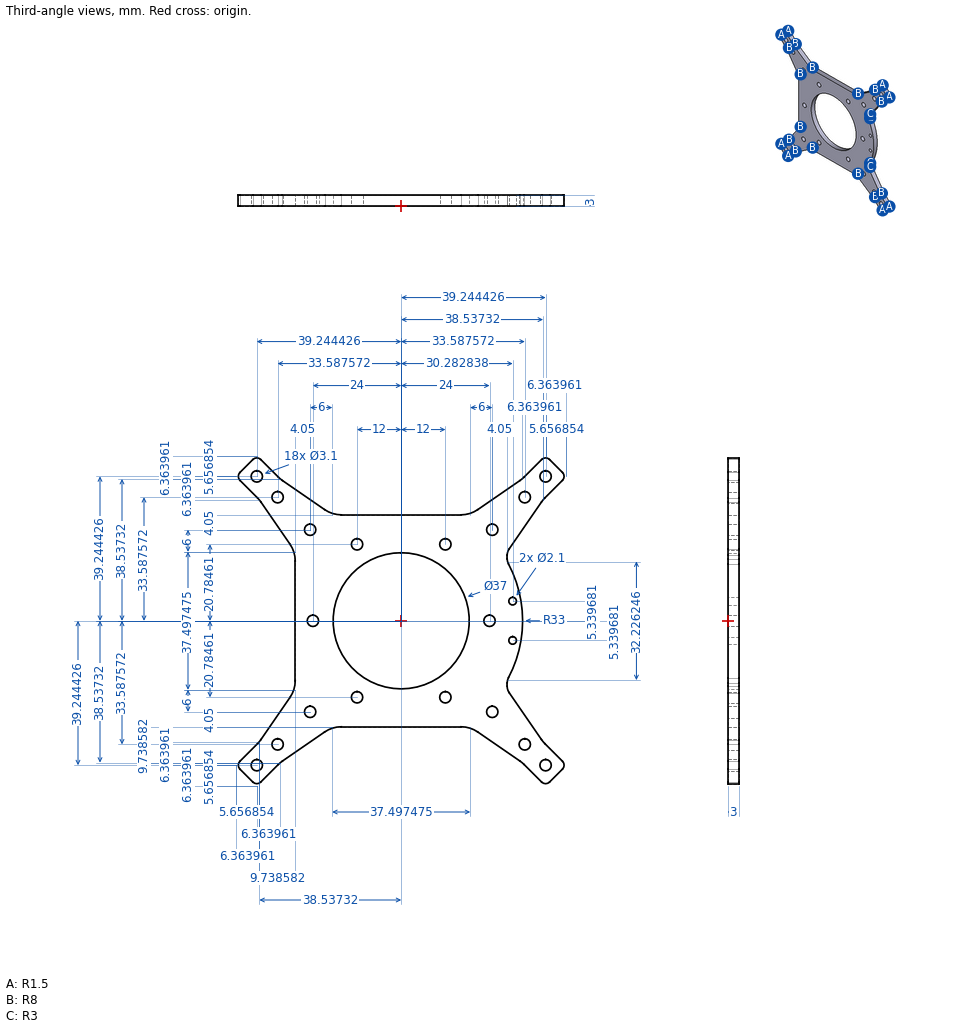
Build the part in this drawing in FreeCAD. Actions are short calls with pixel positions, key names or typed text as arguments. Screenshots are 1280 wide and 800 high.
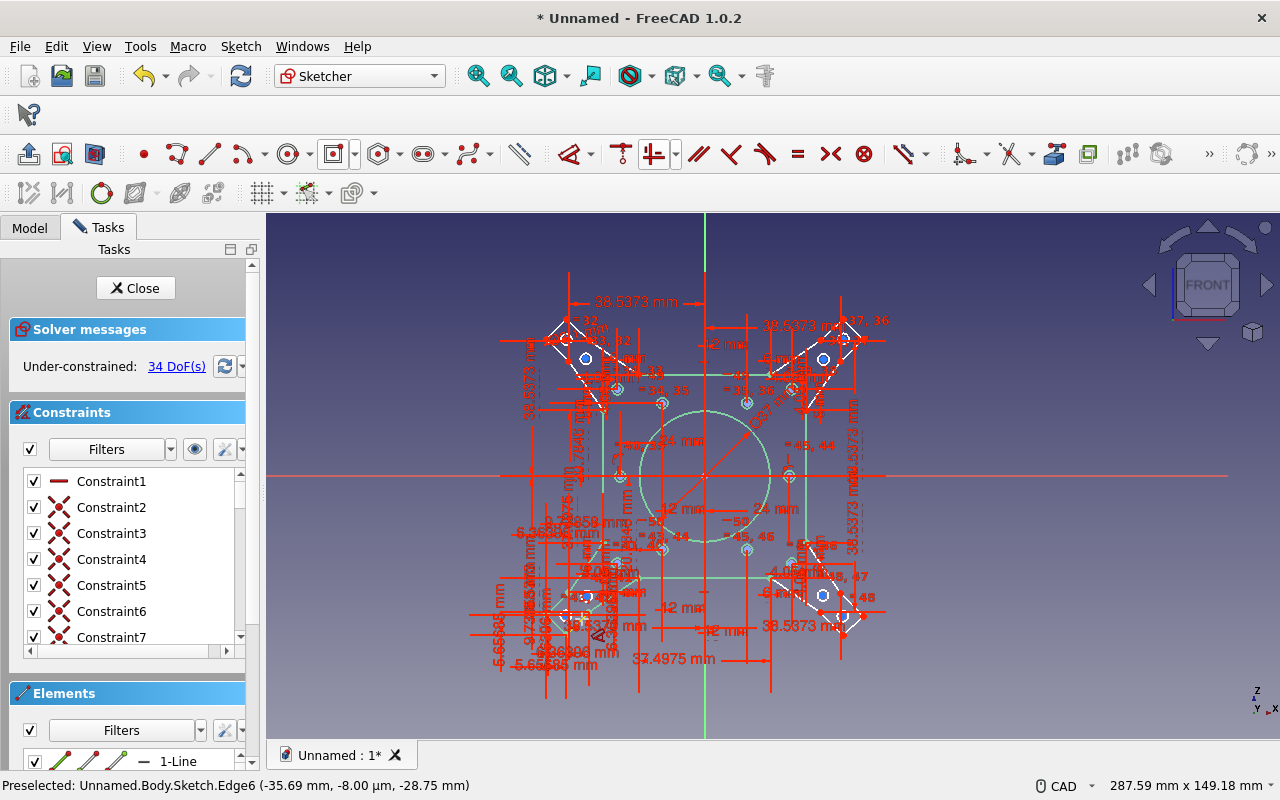
scroll(562, 355, up, 3)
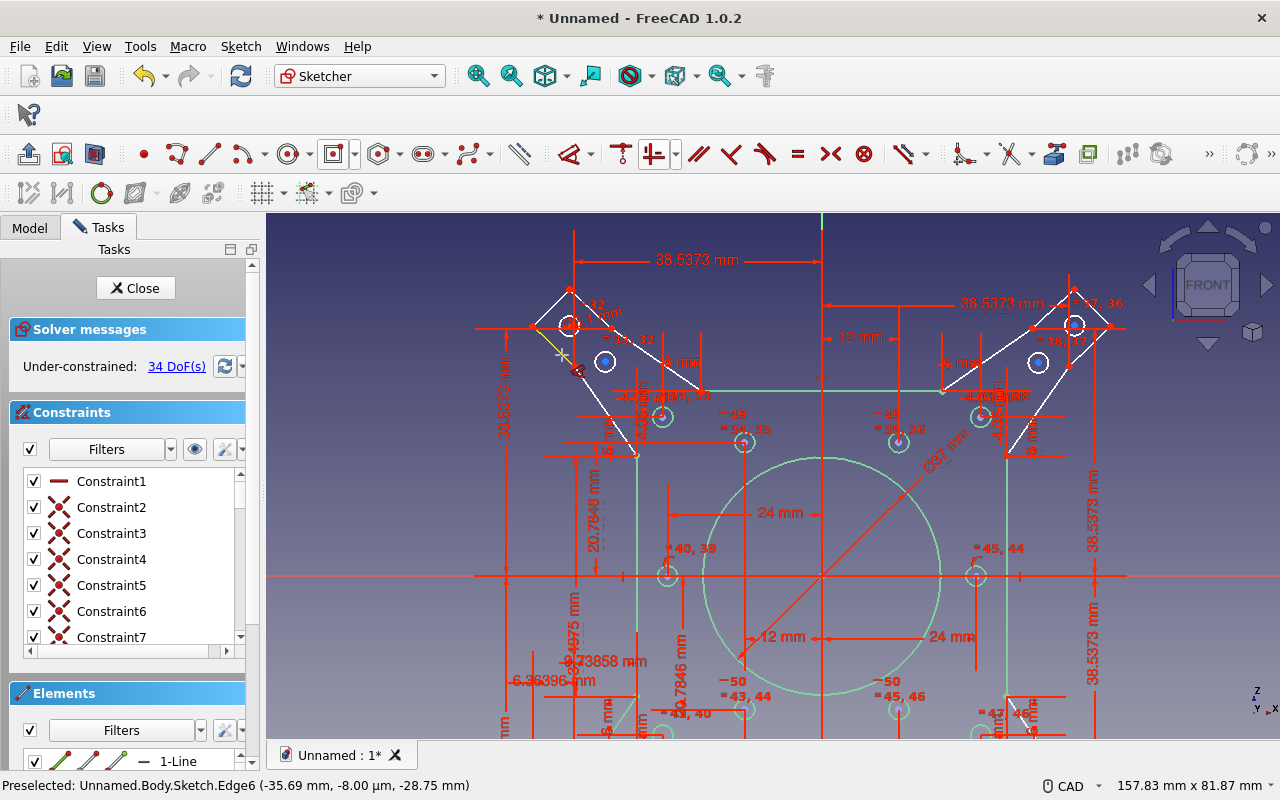
click(562, 354)
click(544, 292)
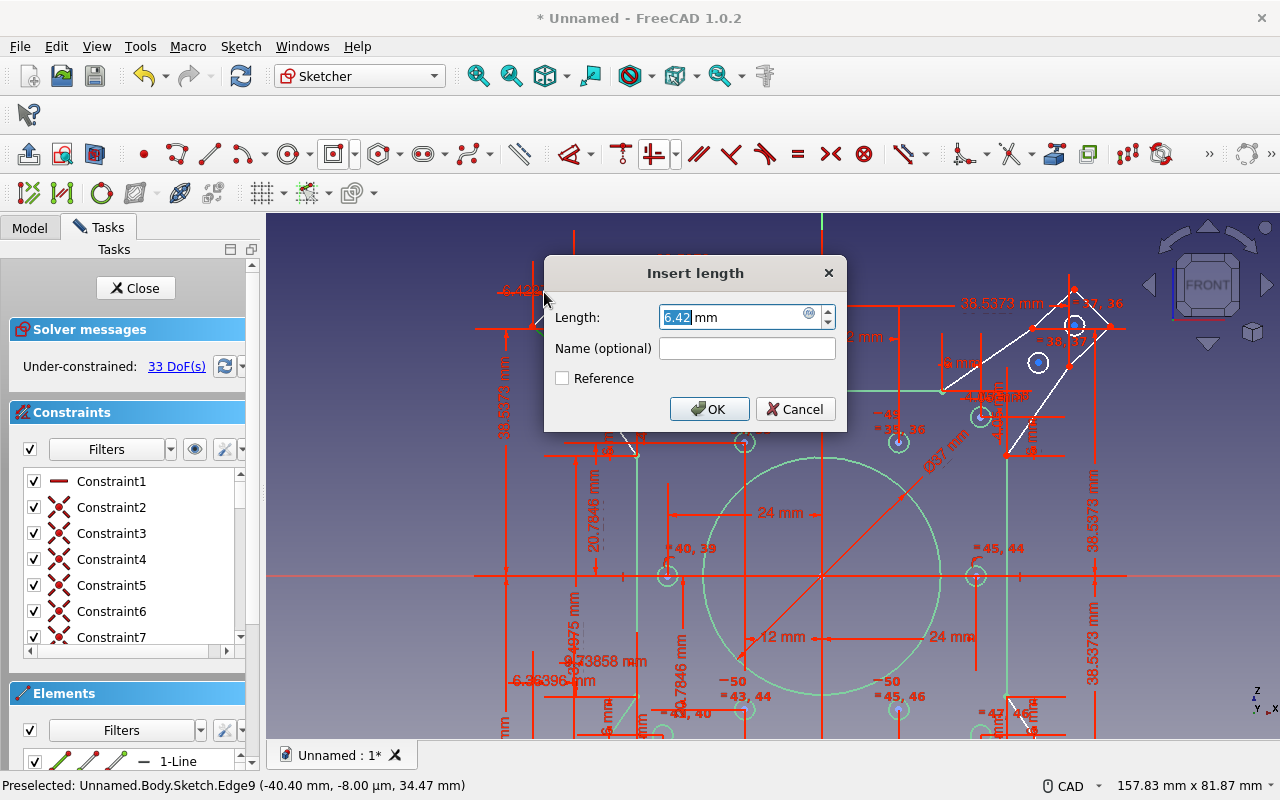
text(6.363961)
key(Return)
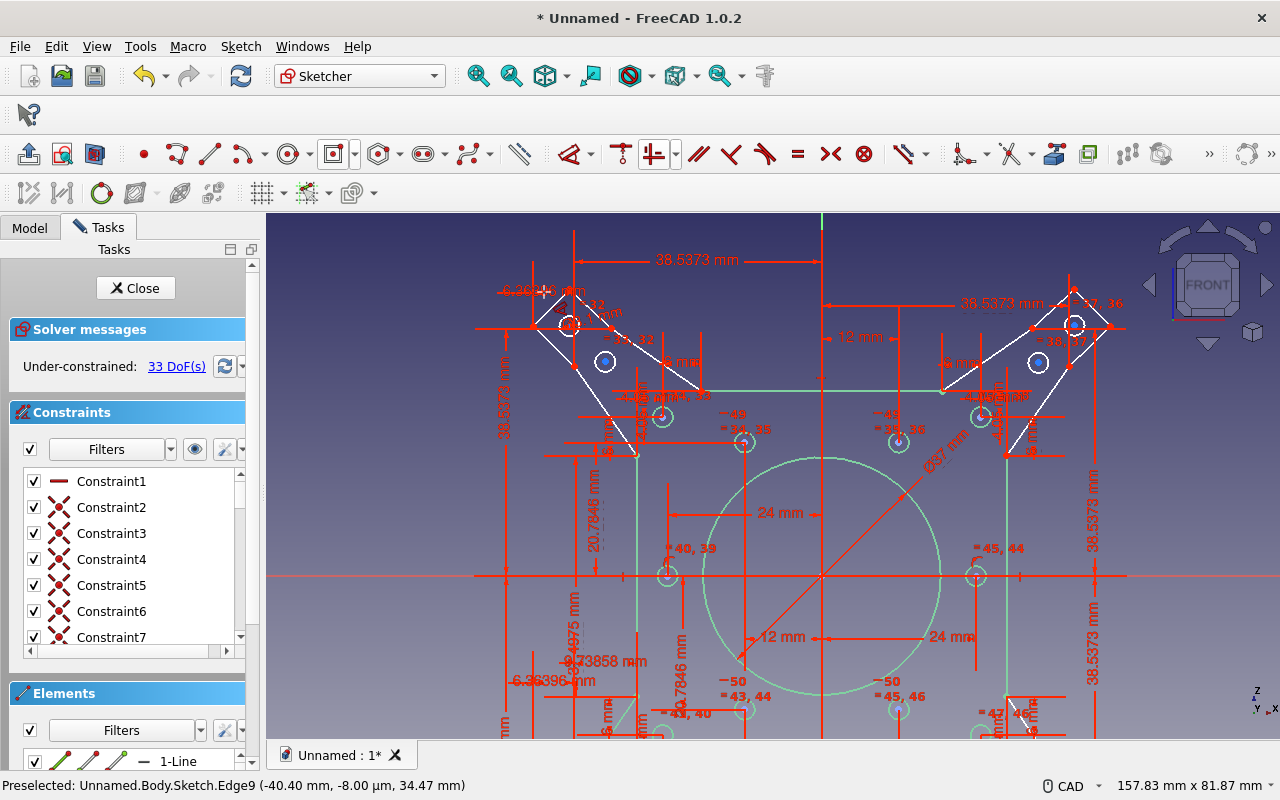
click(562, 354)
click(499, 346)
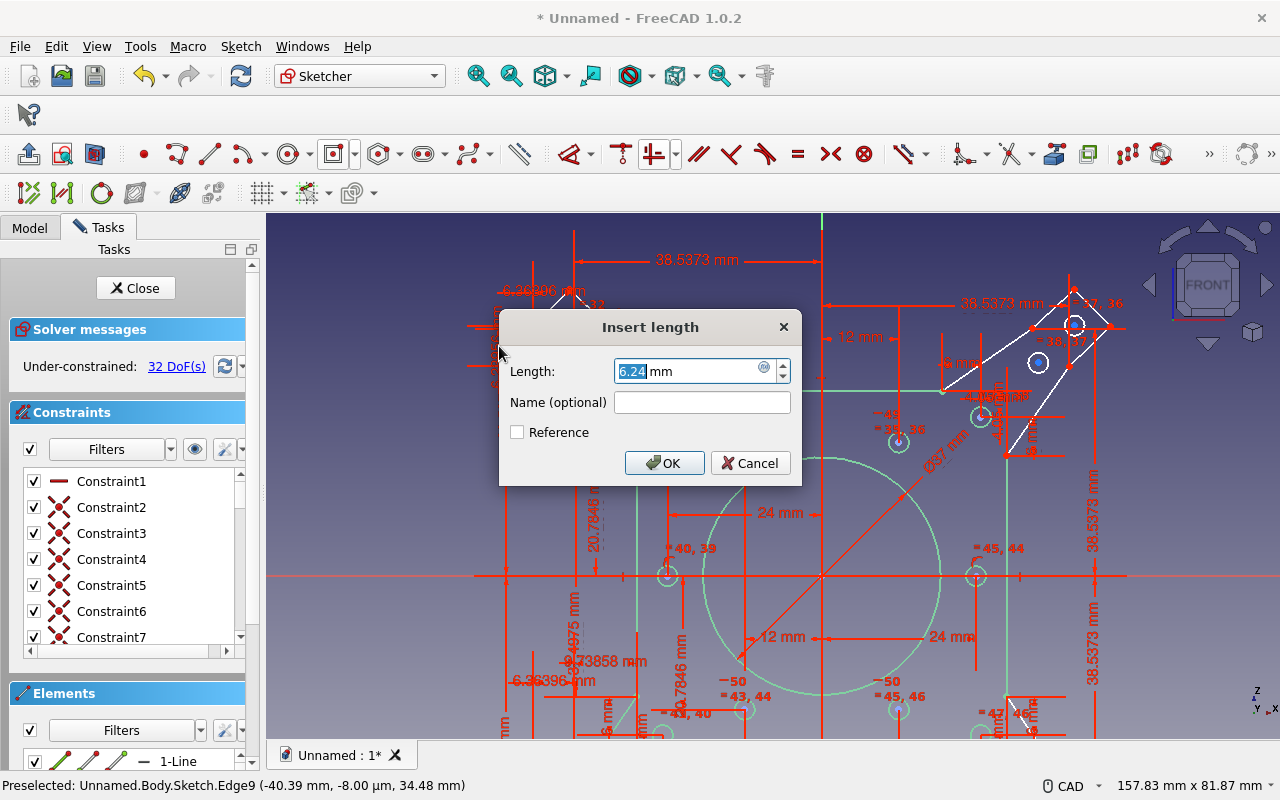
text(6.363961)
key(Return)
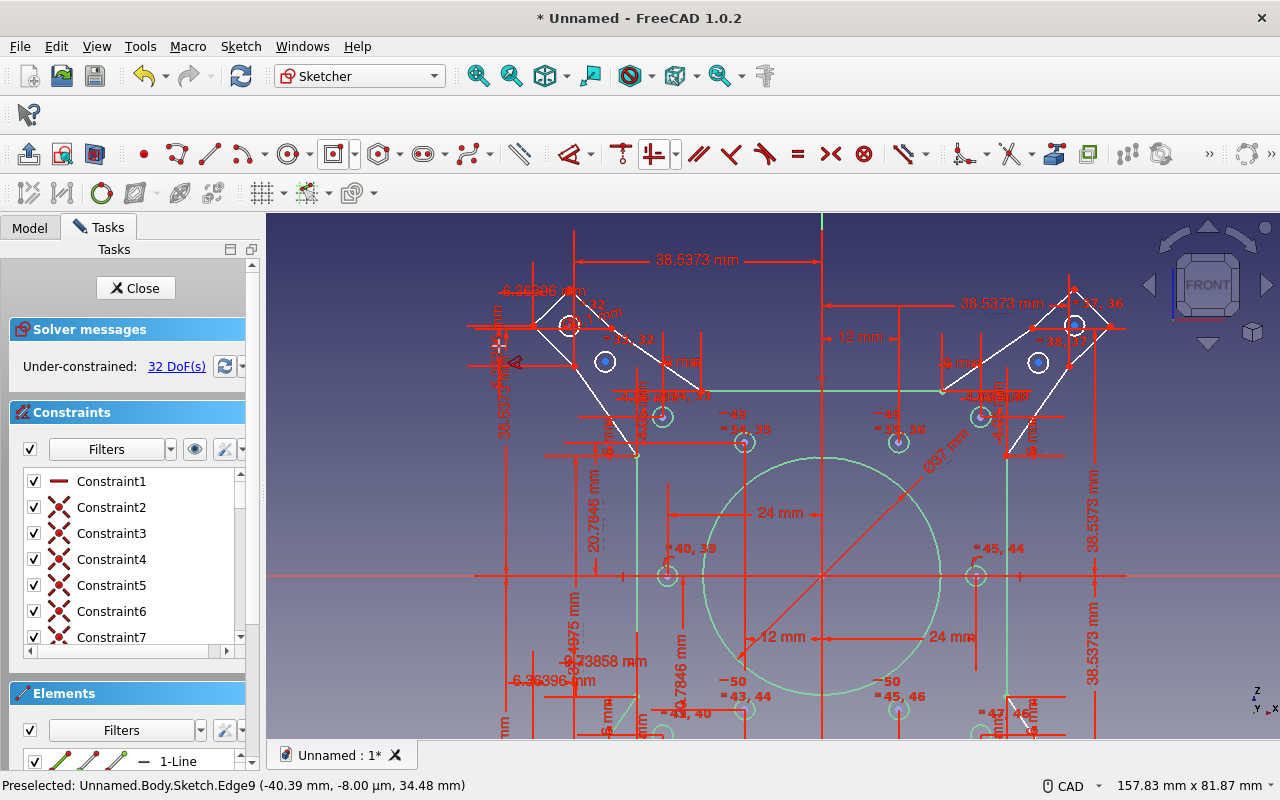
click(544, 315)
click(551, 256)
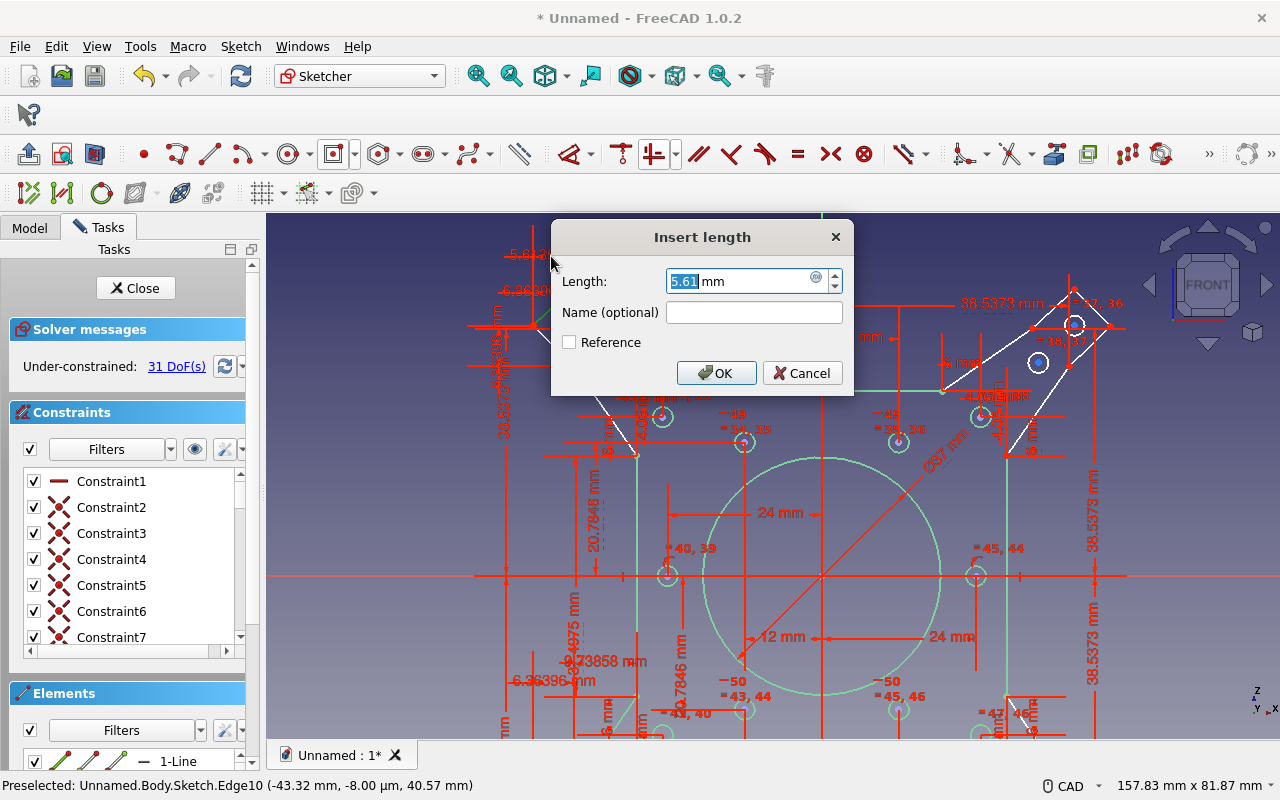
text(5.656854)
key(Return)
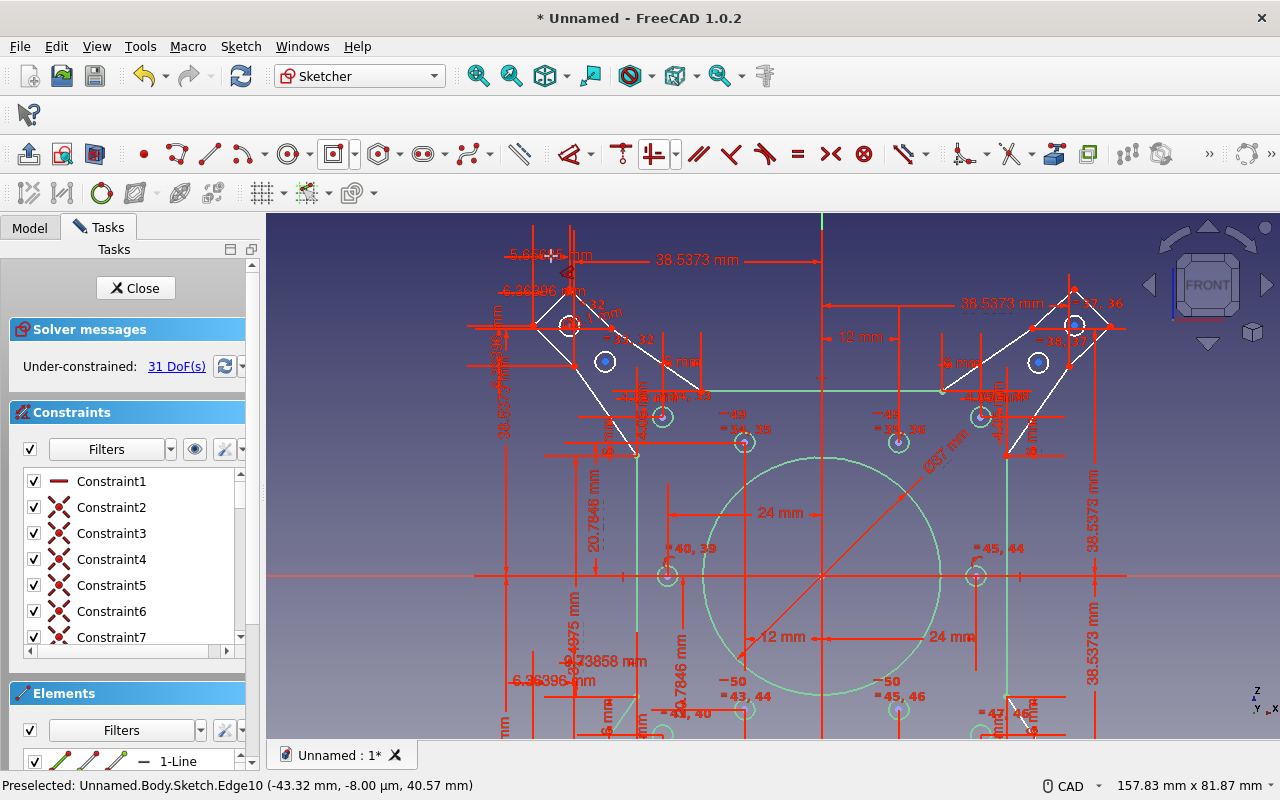
click(544, 315)
click(499, 316)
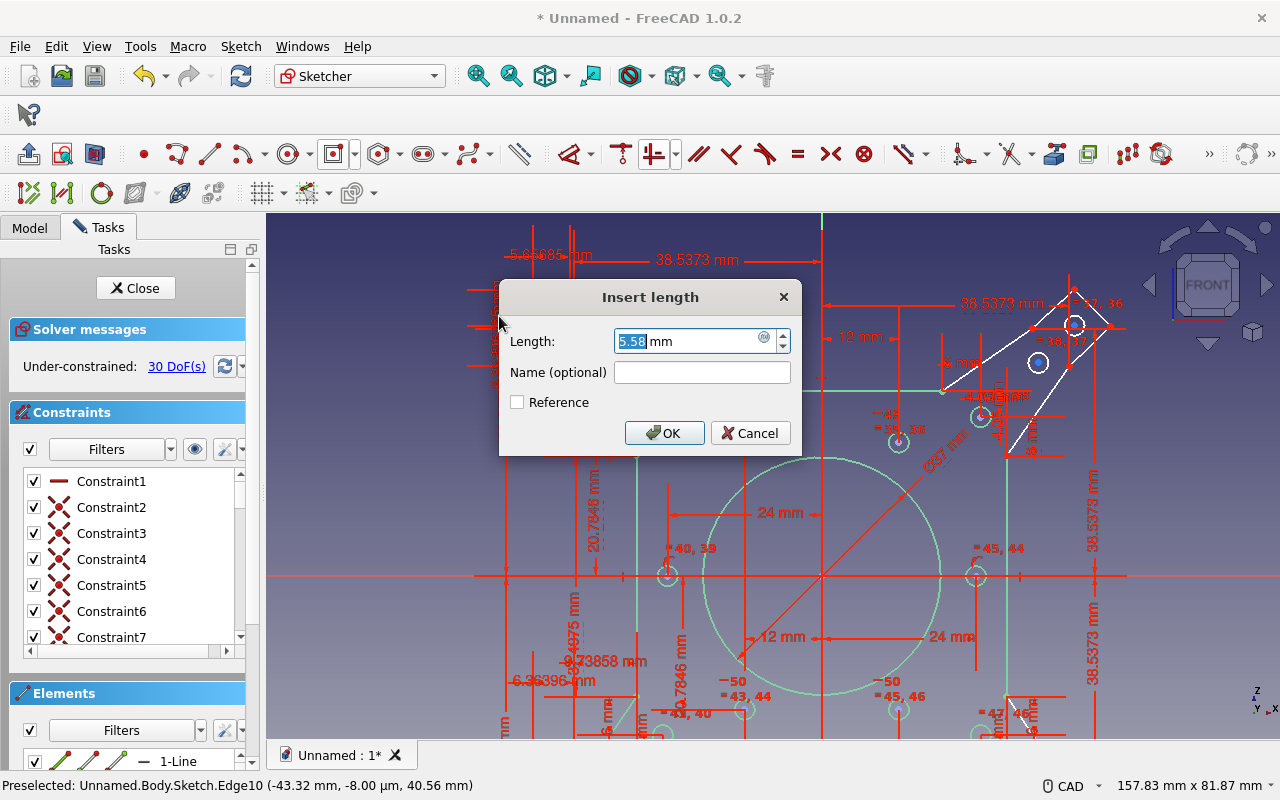
text(5.656854)
key(Return)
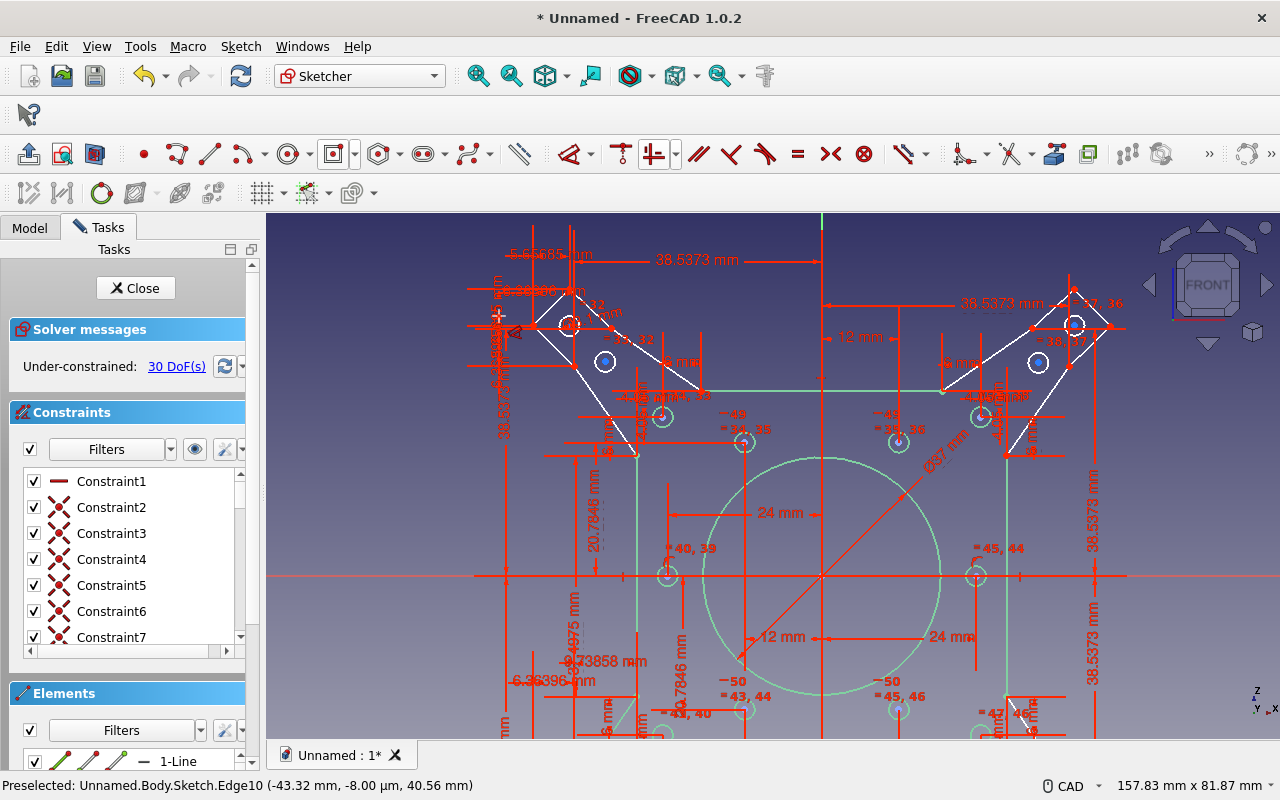
click(582, 301)
click(591, 459)